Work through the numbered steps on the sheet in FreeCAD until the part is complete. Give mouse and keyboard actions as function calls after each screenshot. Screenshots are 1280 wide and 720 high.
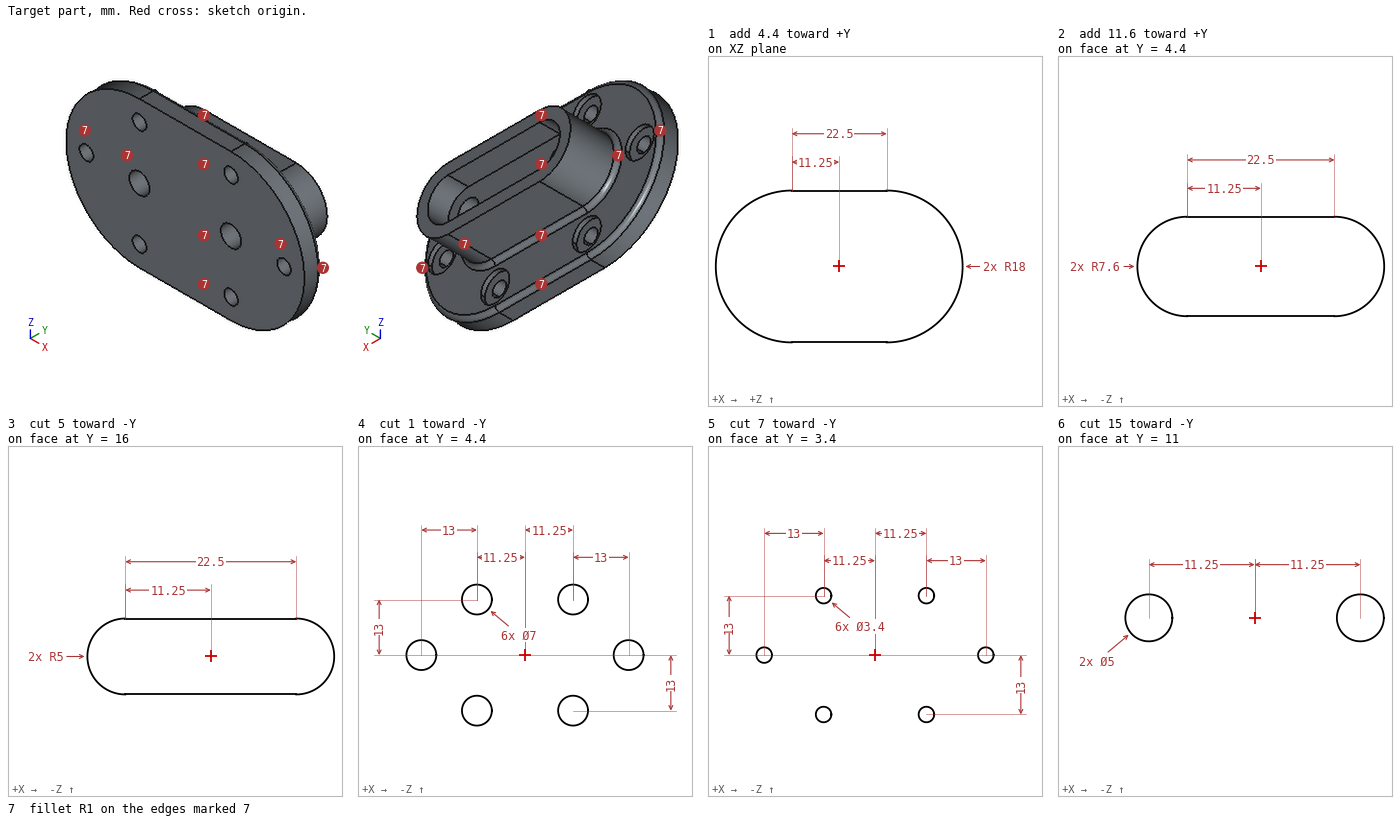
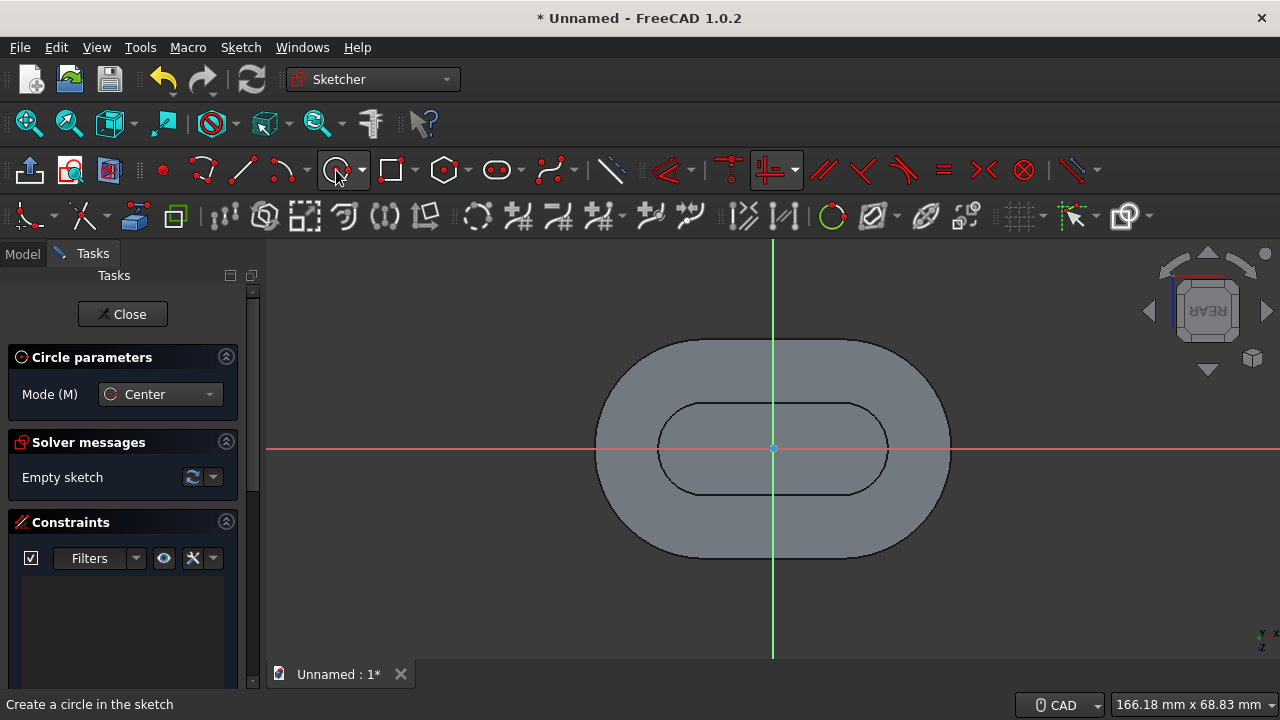
click(704, 370)
move(719, 355)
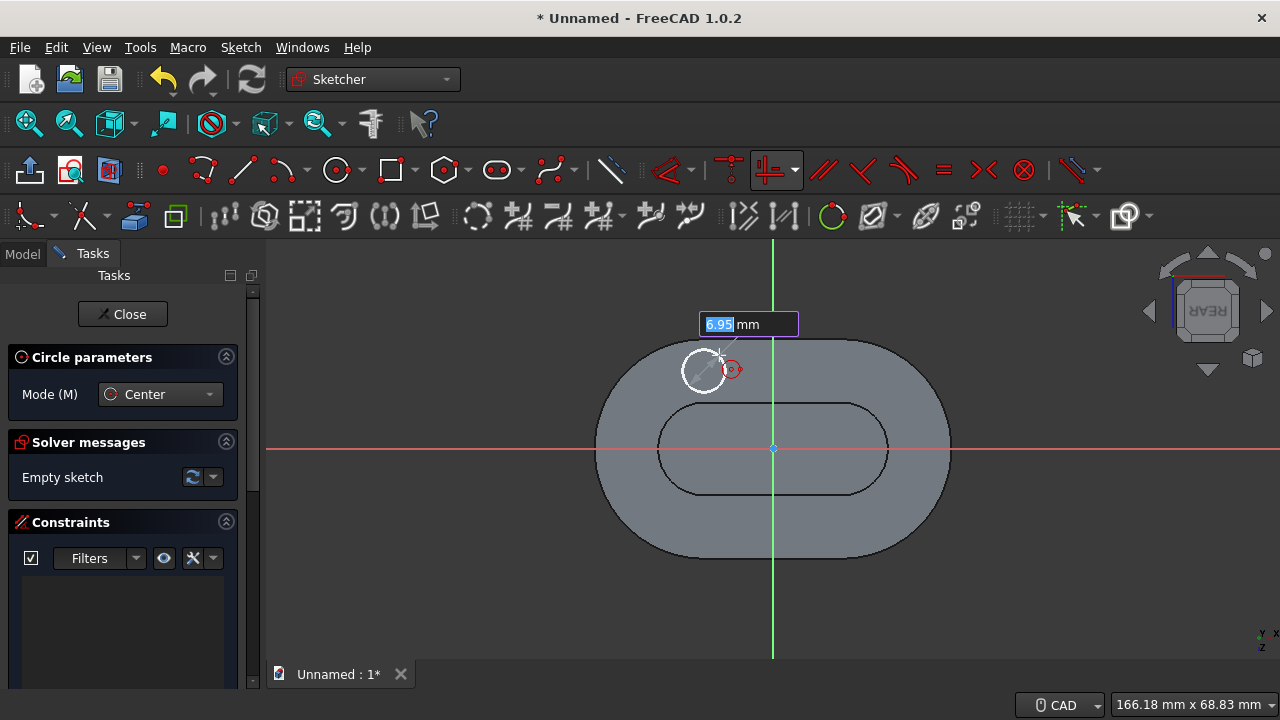
text(7)
key(Return)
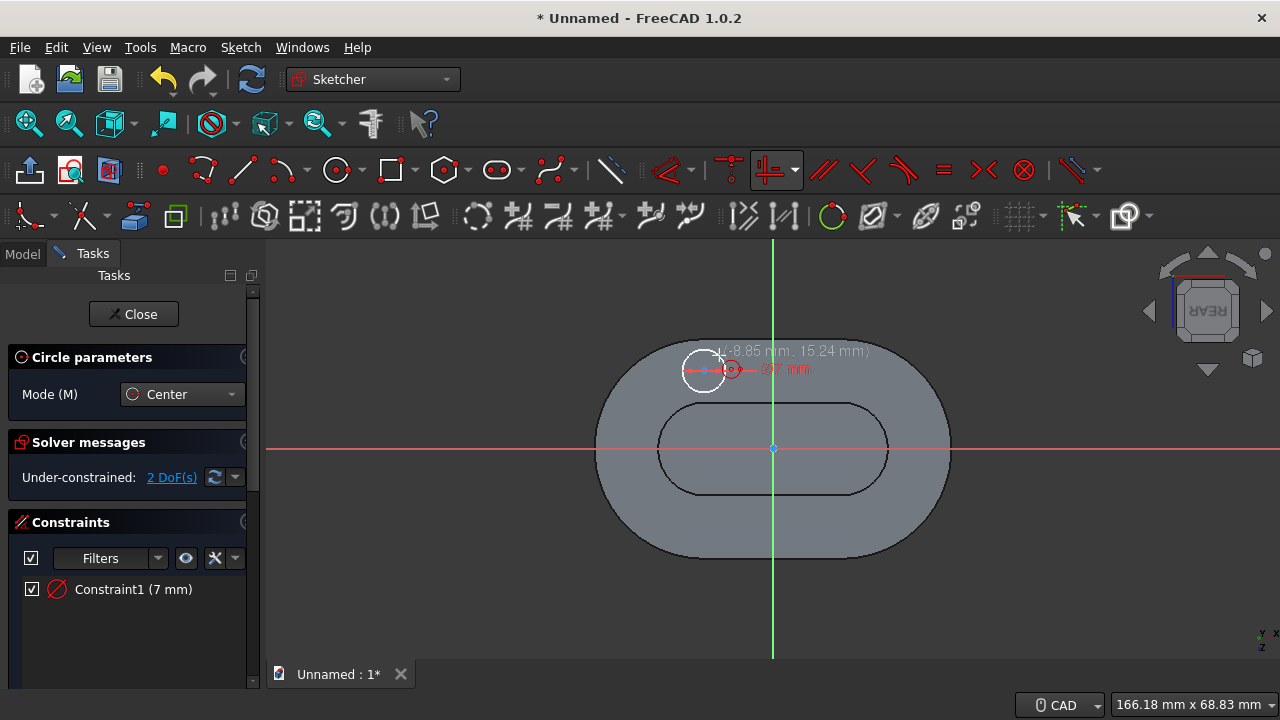
click(842, 370)
move(857, 355)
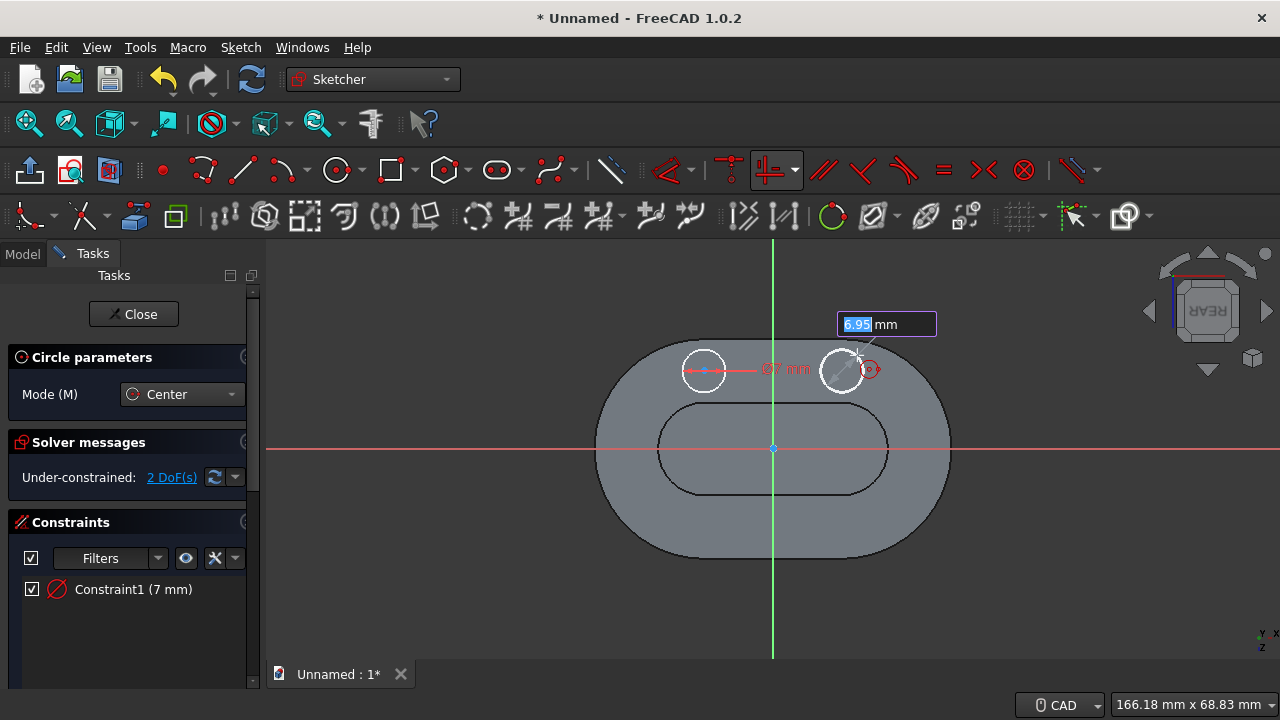
text(7)
key(Return)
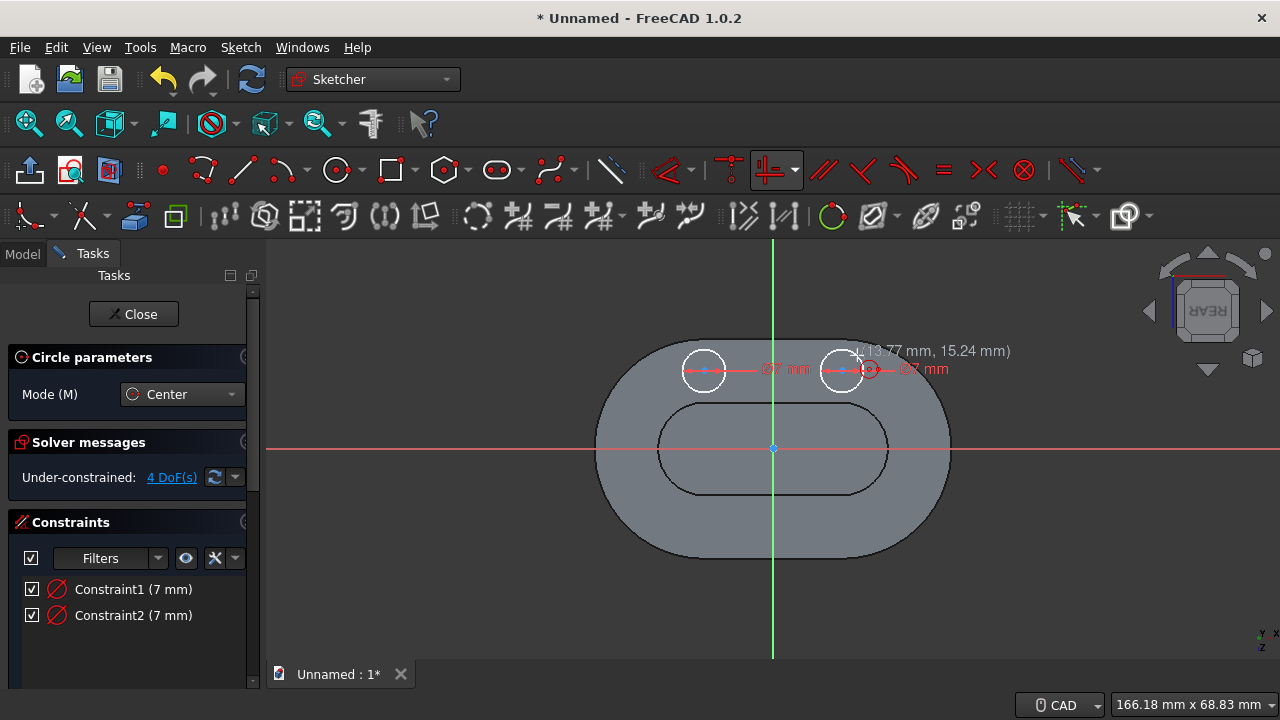
click(842, 528)
move(857, 513)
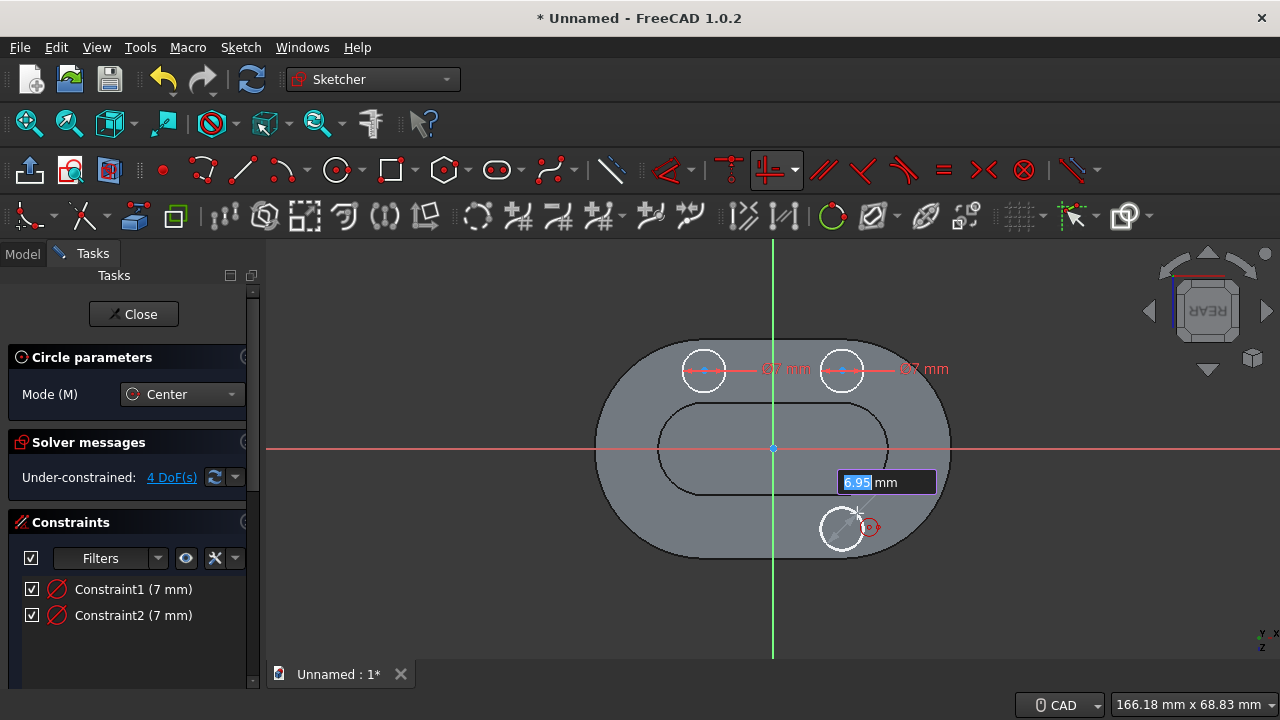
text(7)
key(Return)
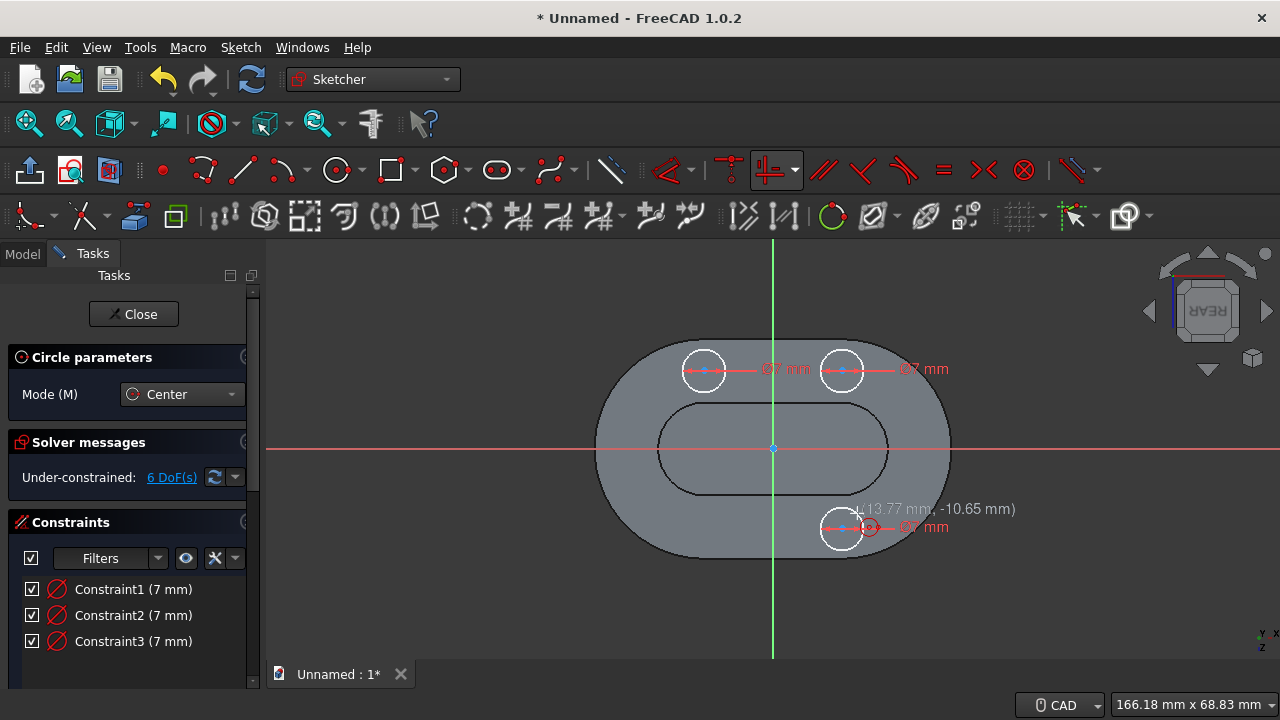
click(704, 528)
move(719, 513)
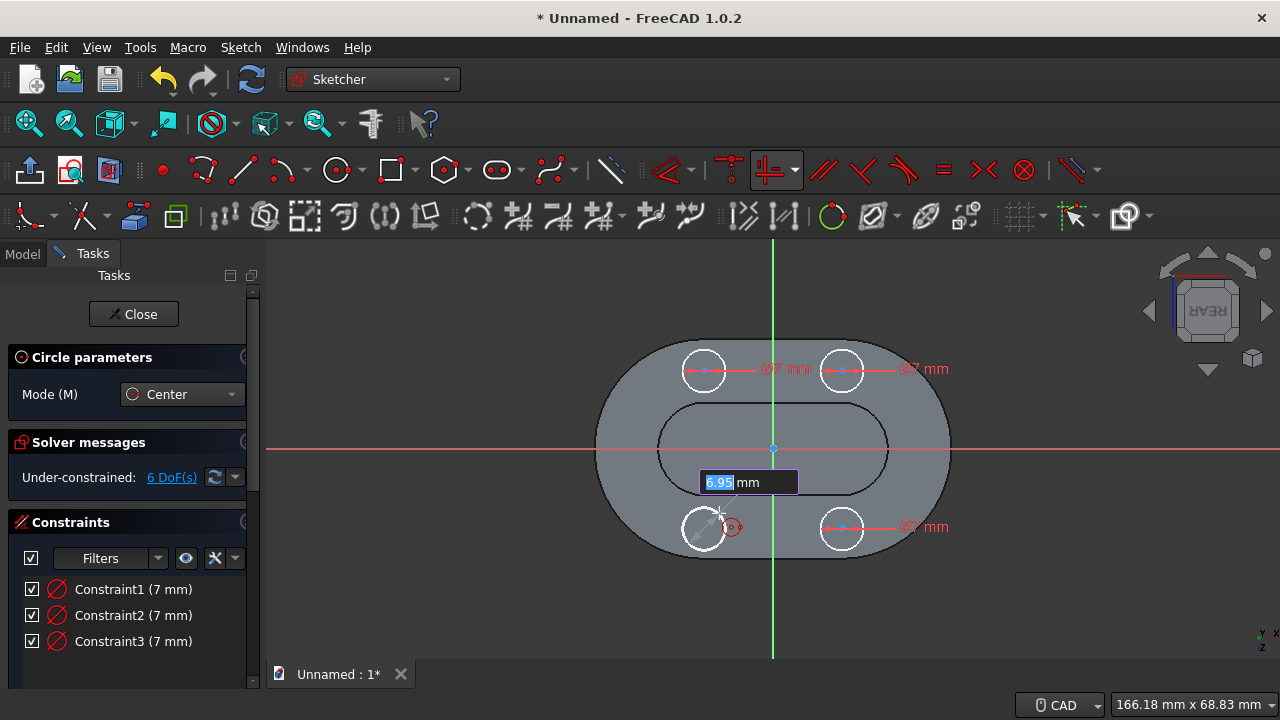
text(7)
key(Return)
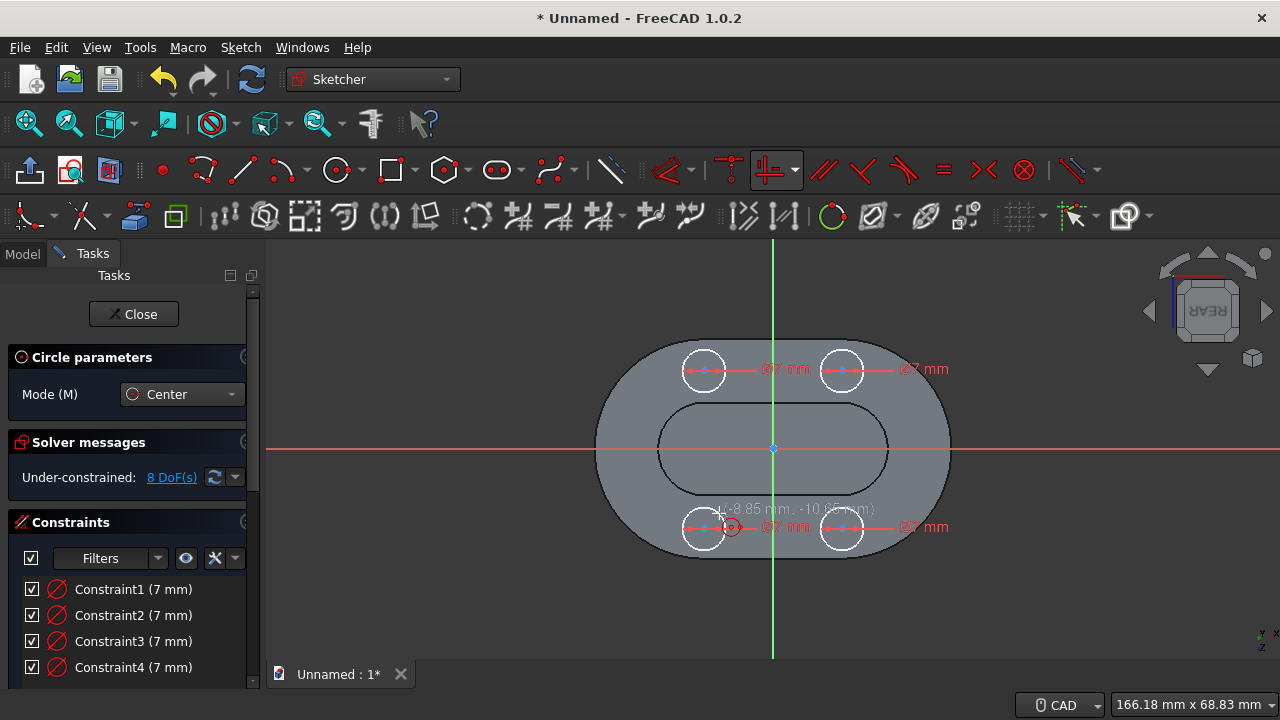
click(625, 449)
move(640, 434)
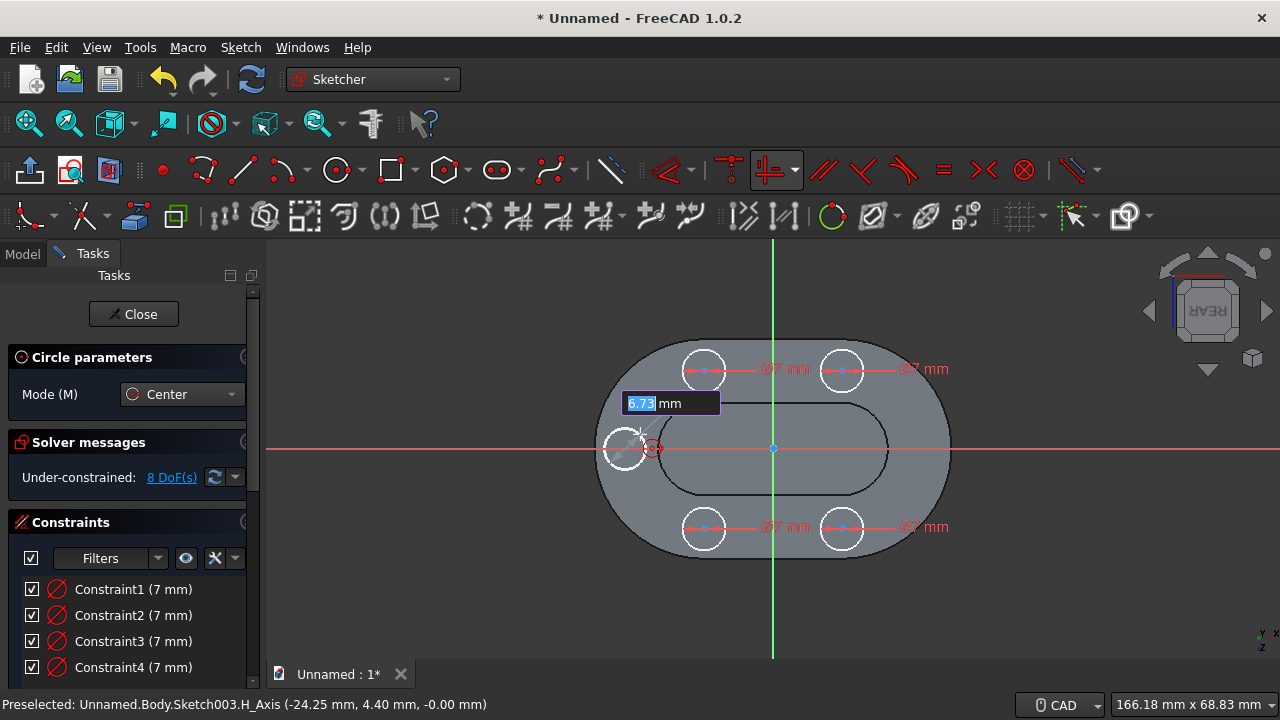
text(7)
key(Return)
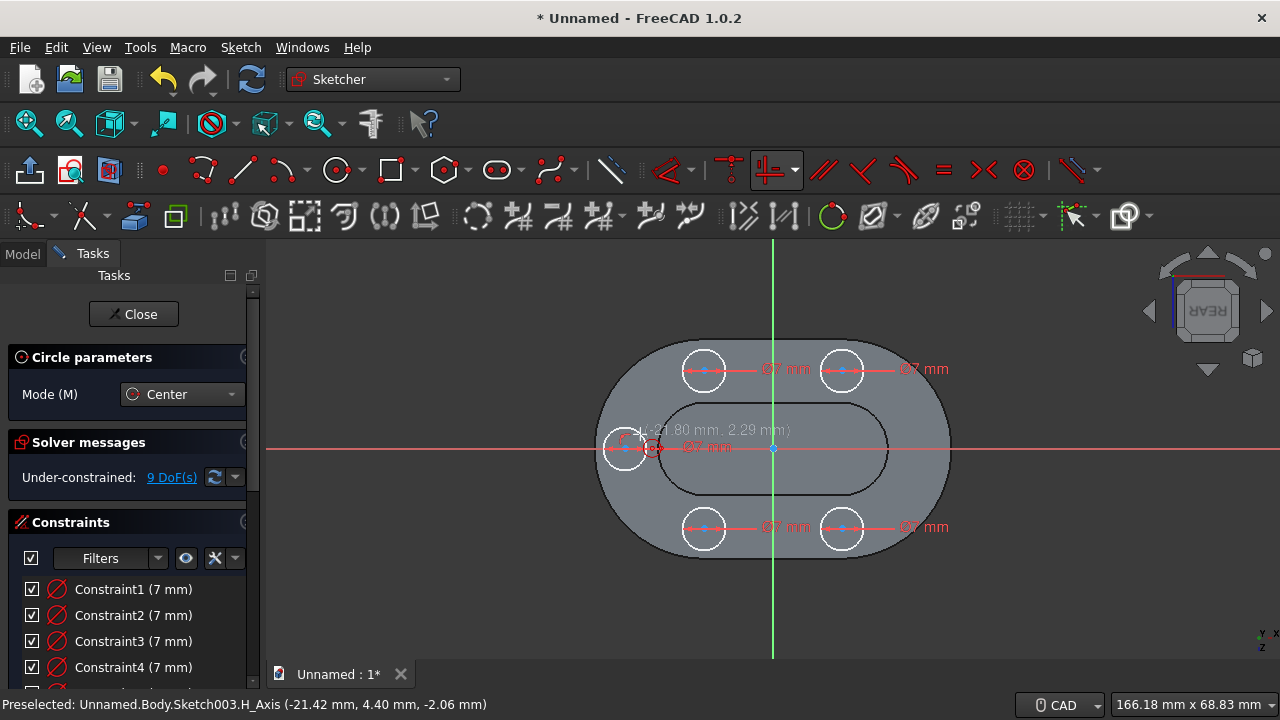
click(921, 449)
move(936, 434)